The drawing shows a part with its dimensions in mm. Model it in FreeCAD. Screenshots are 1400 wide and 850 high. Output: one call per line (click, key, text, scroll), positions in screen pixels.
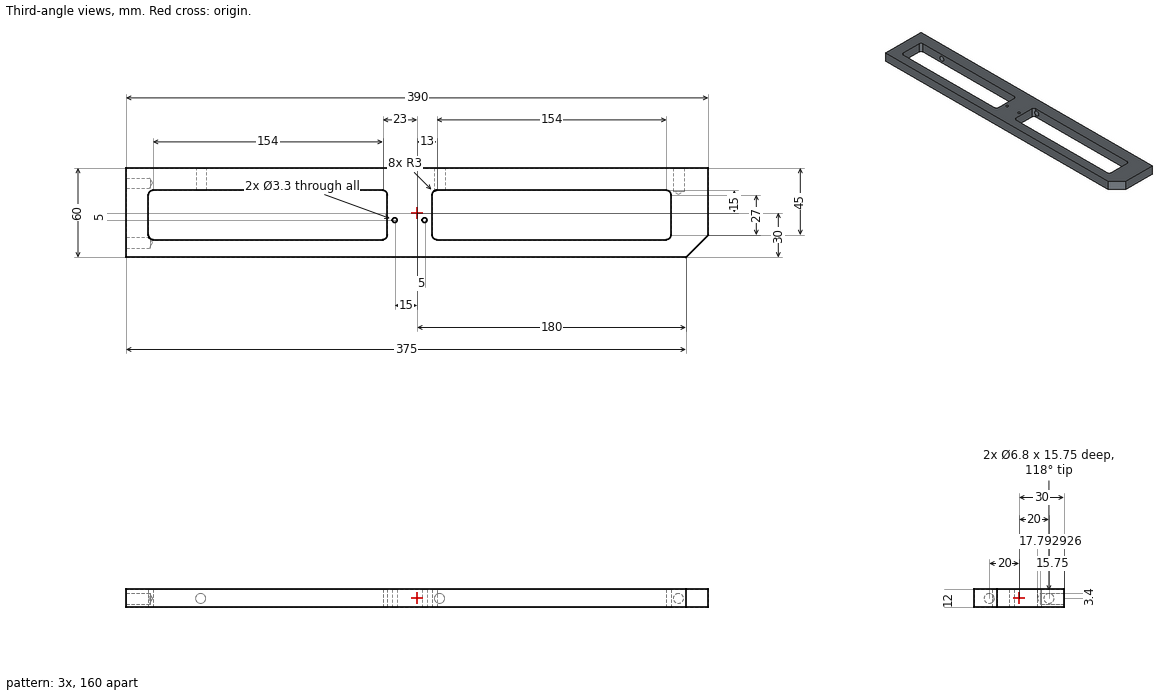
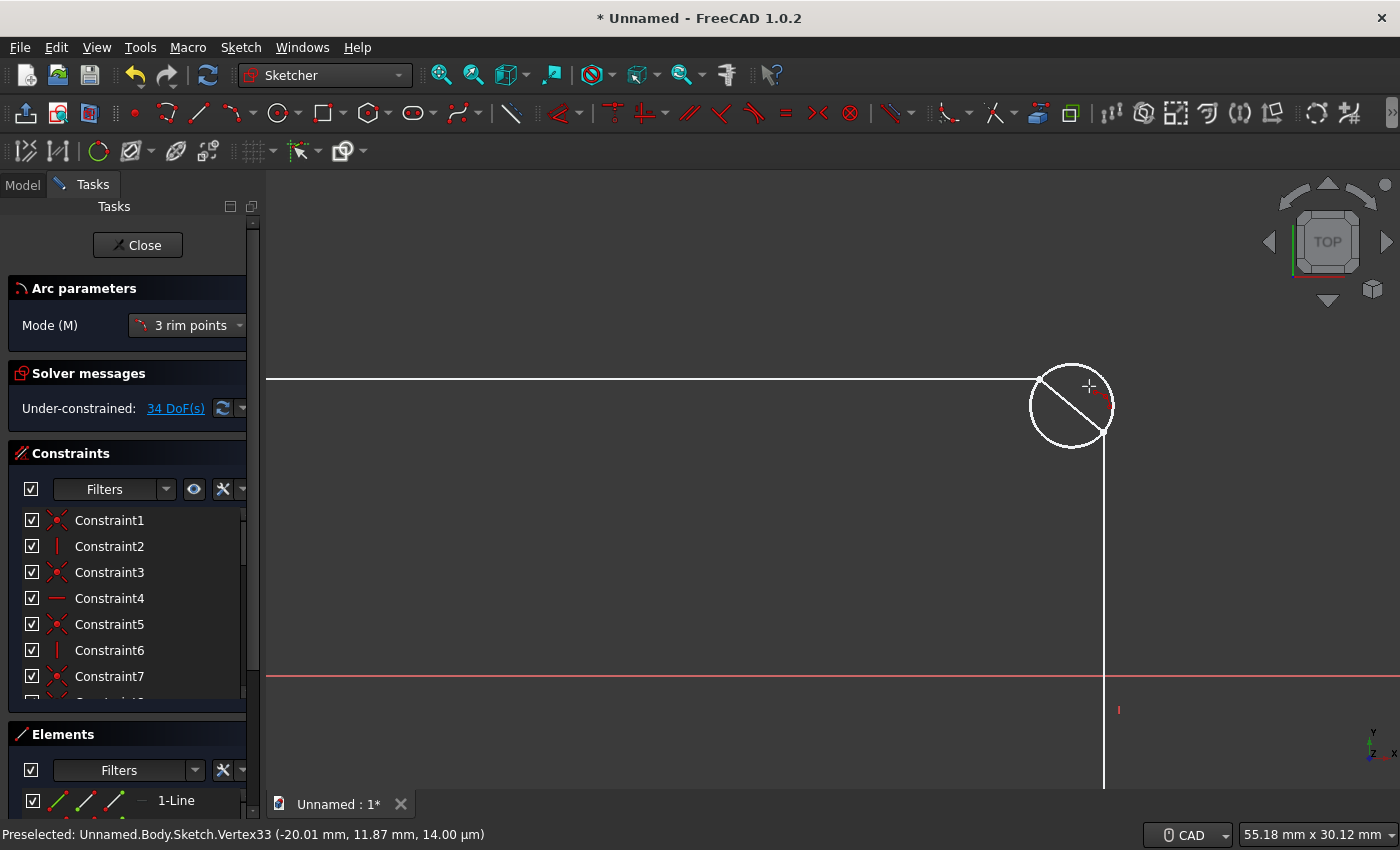
click(1086, 386)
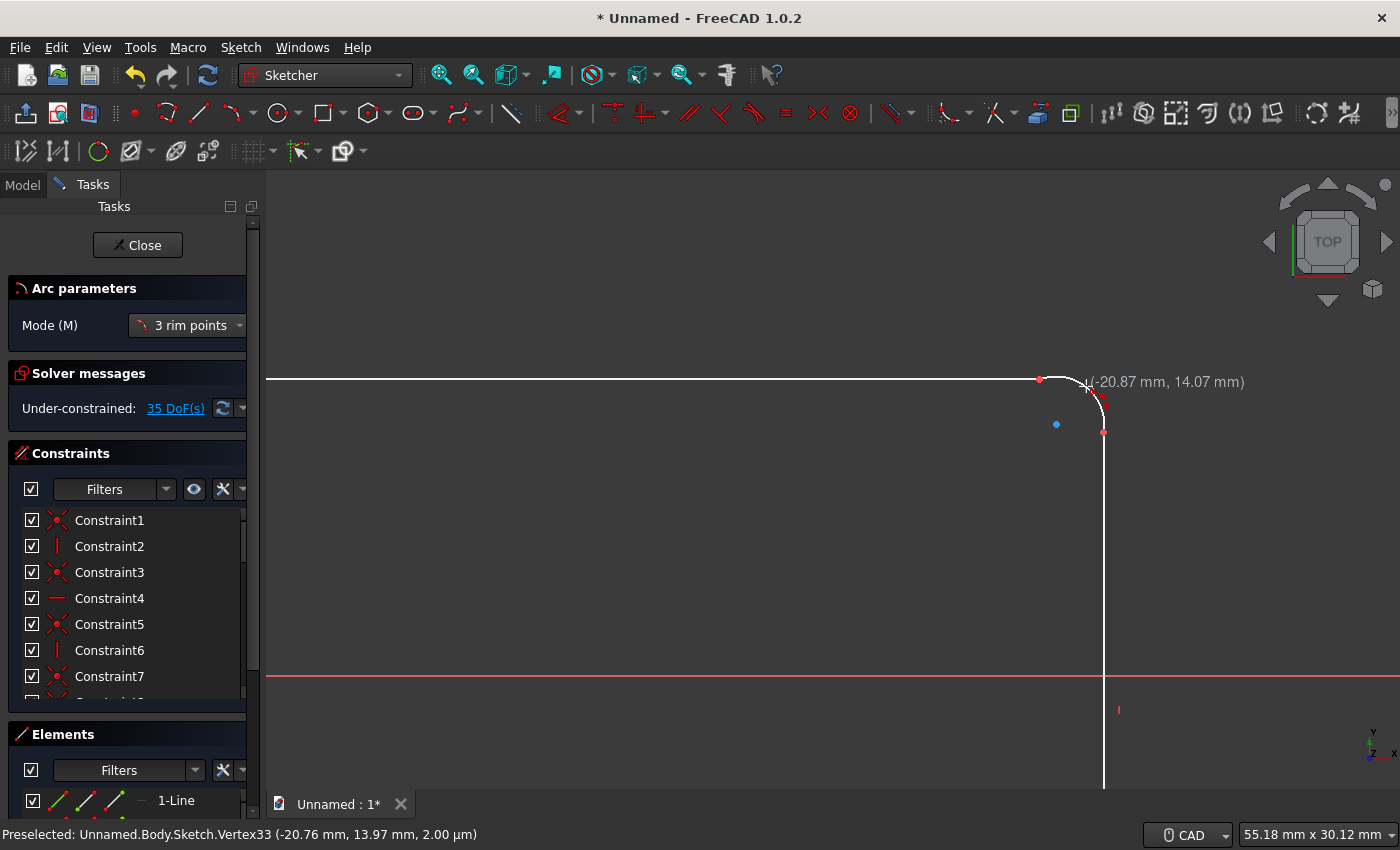
scroll(690, 460, down, 12)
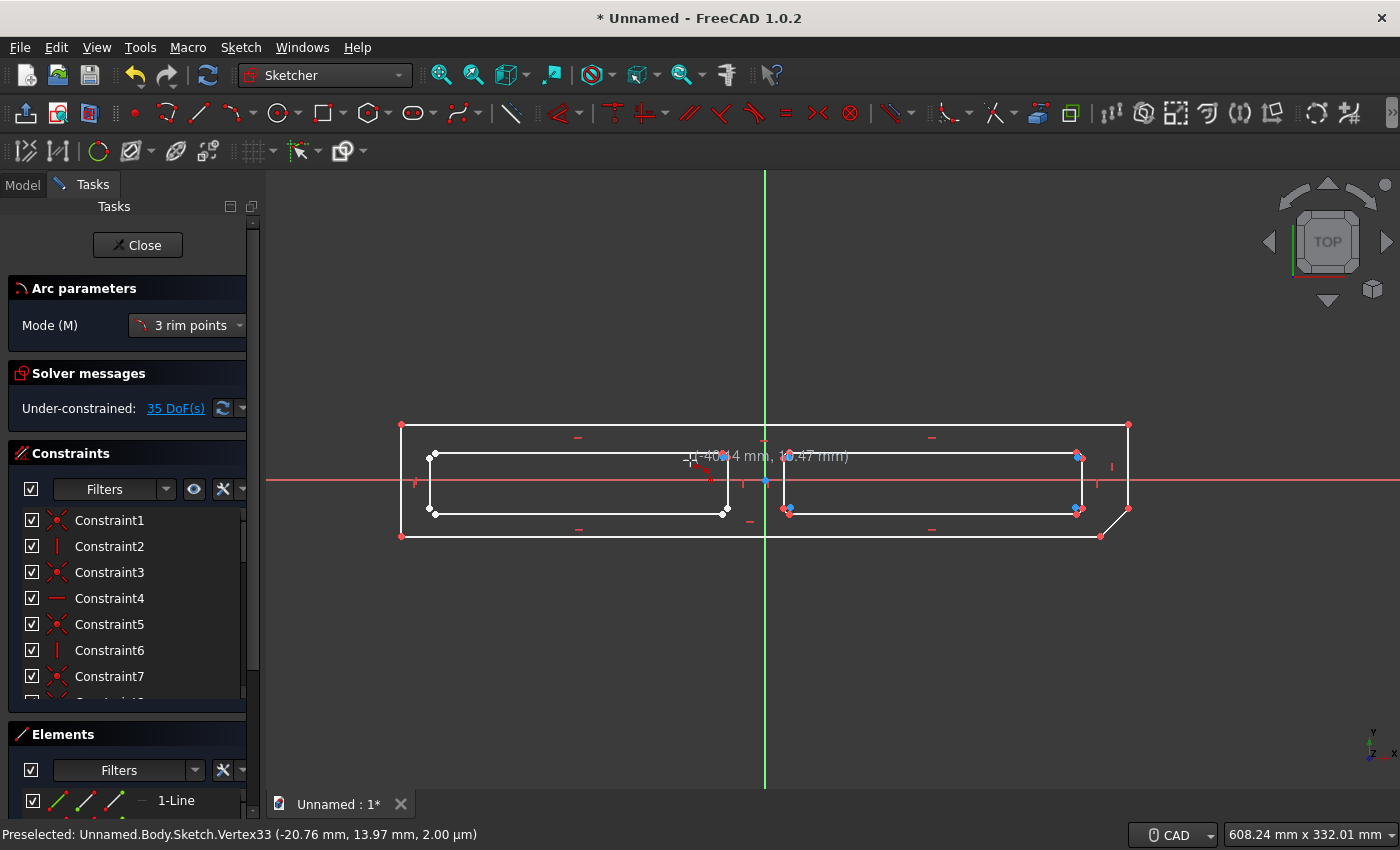
scroll(728, 508, up, 4)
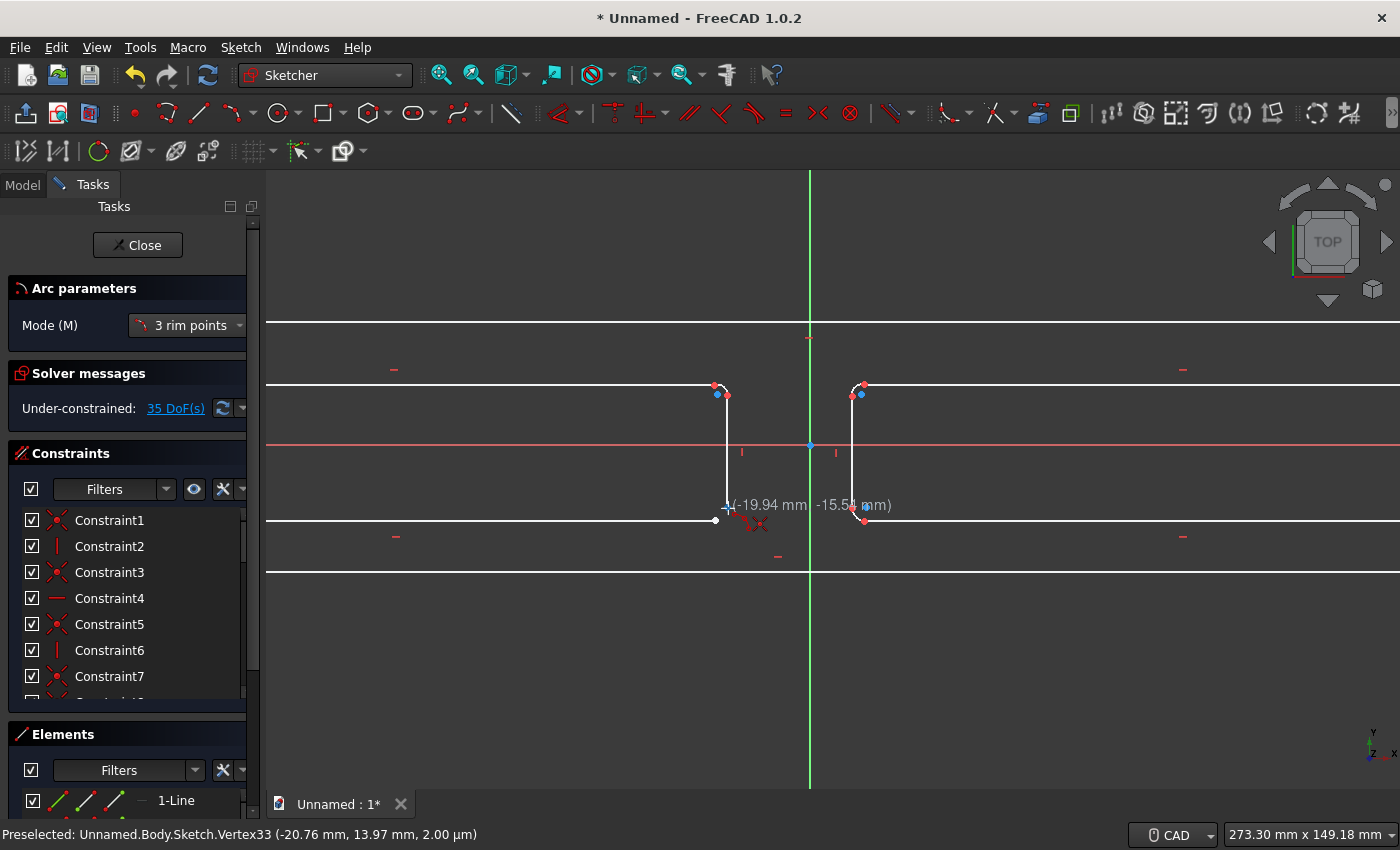
click(727, 508)
click(715, 521)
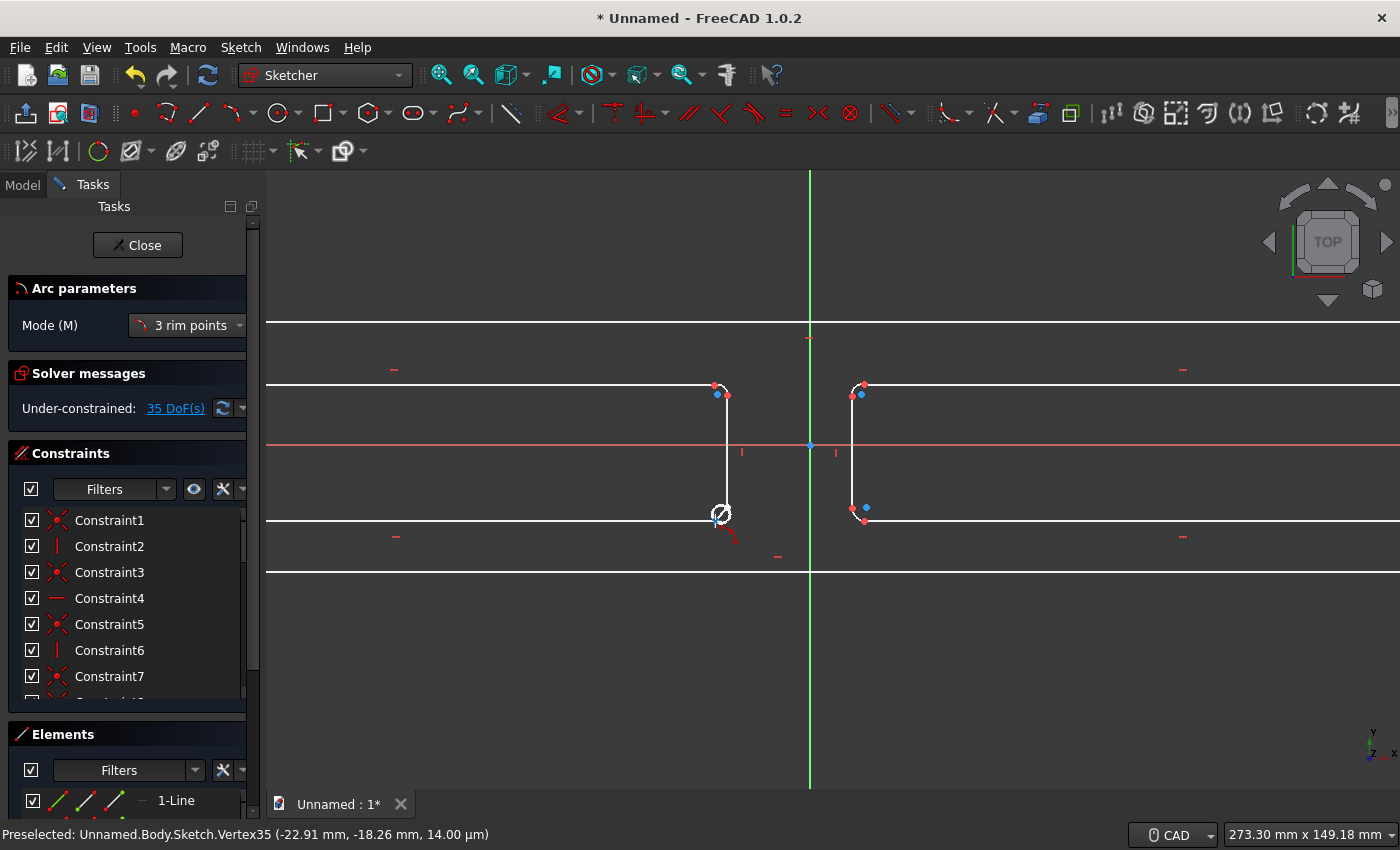
scroll(724, 516, up, 8)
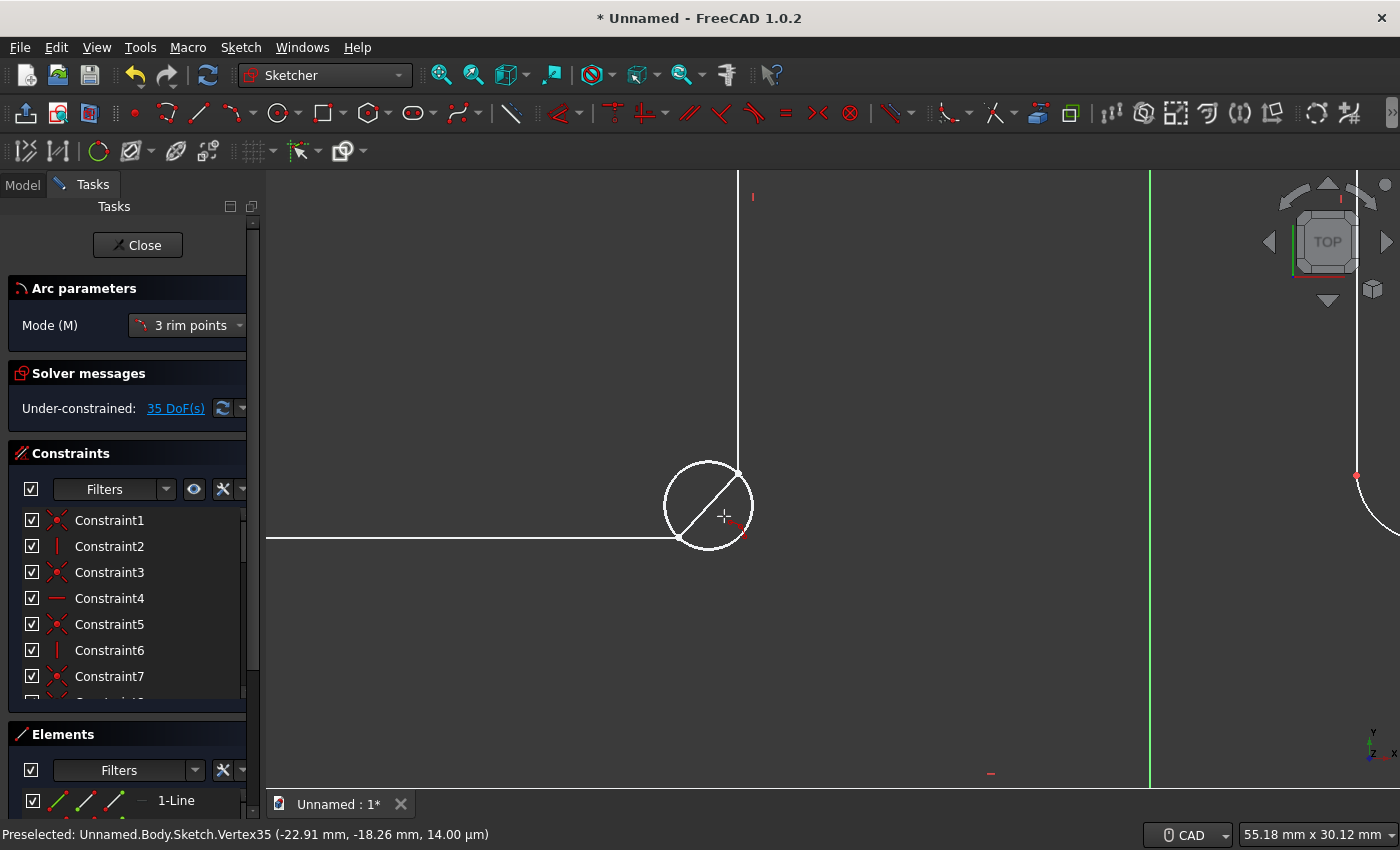
click(720, 514)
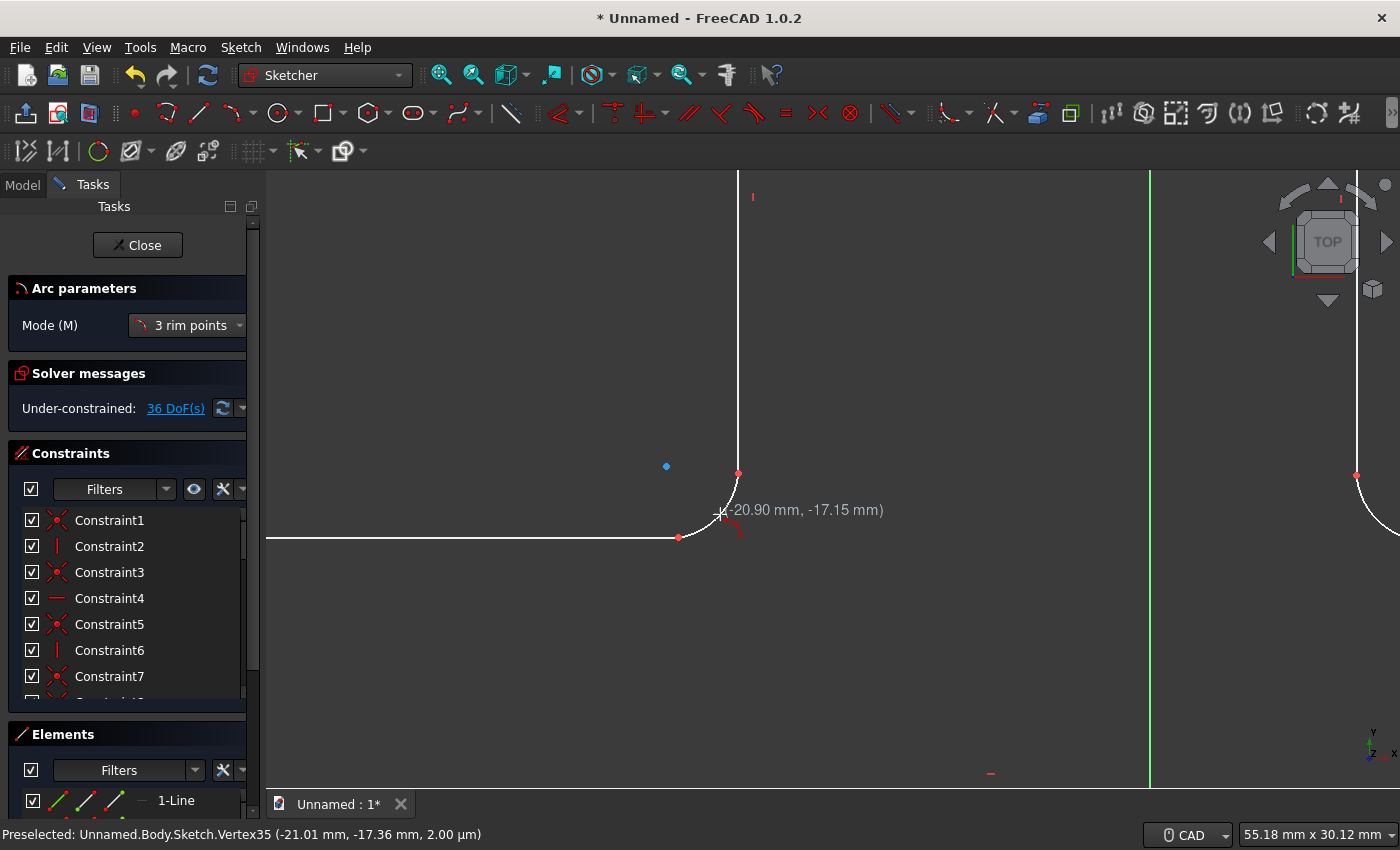
scroll(726, 511, down, 12)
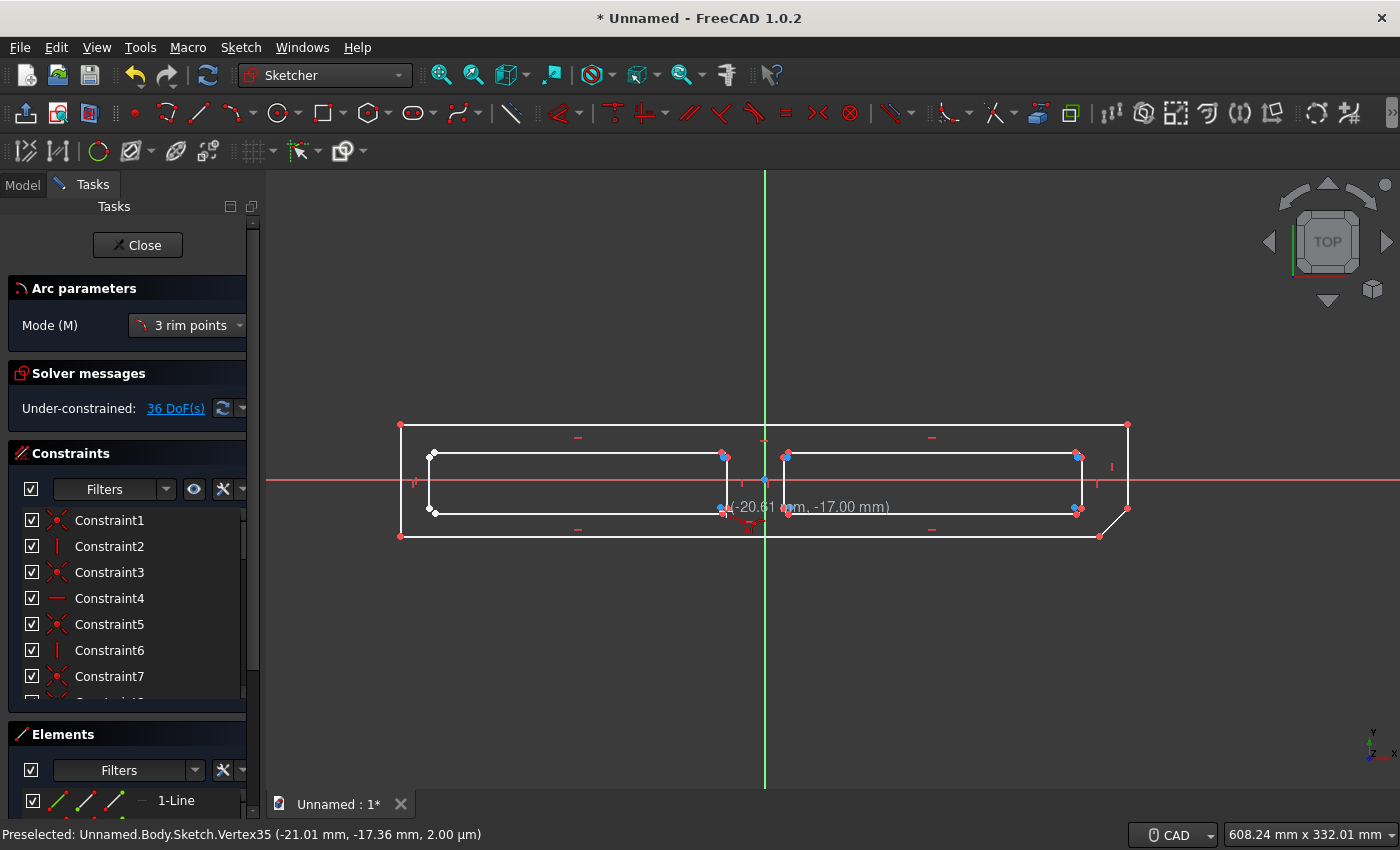
scroll(435, 513, up, 4)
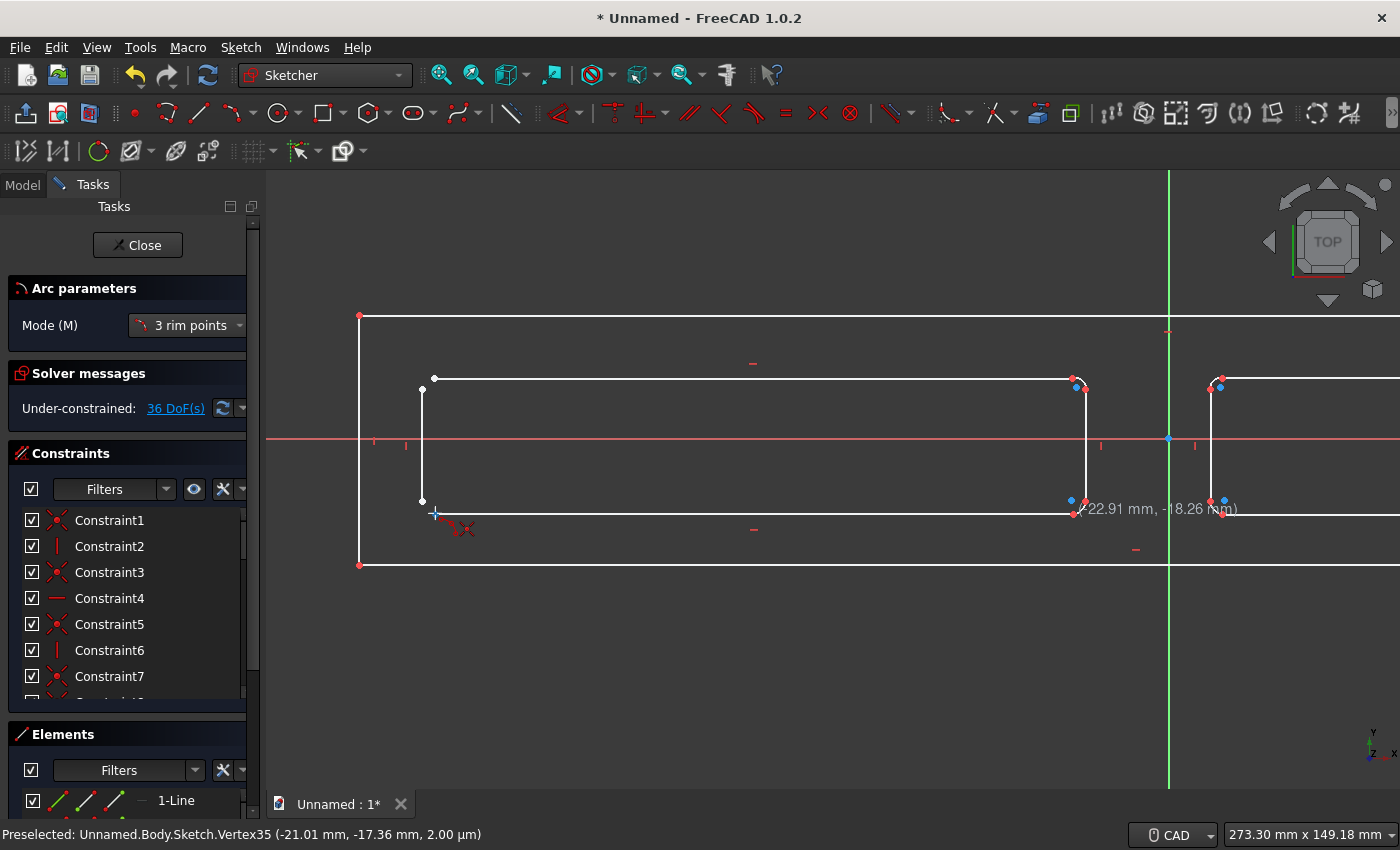
click(435, 514)
click(422, 502)